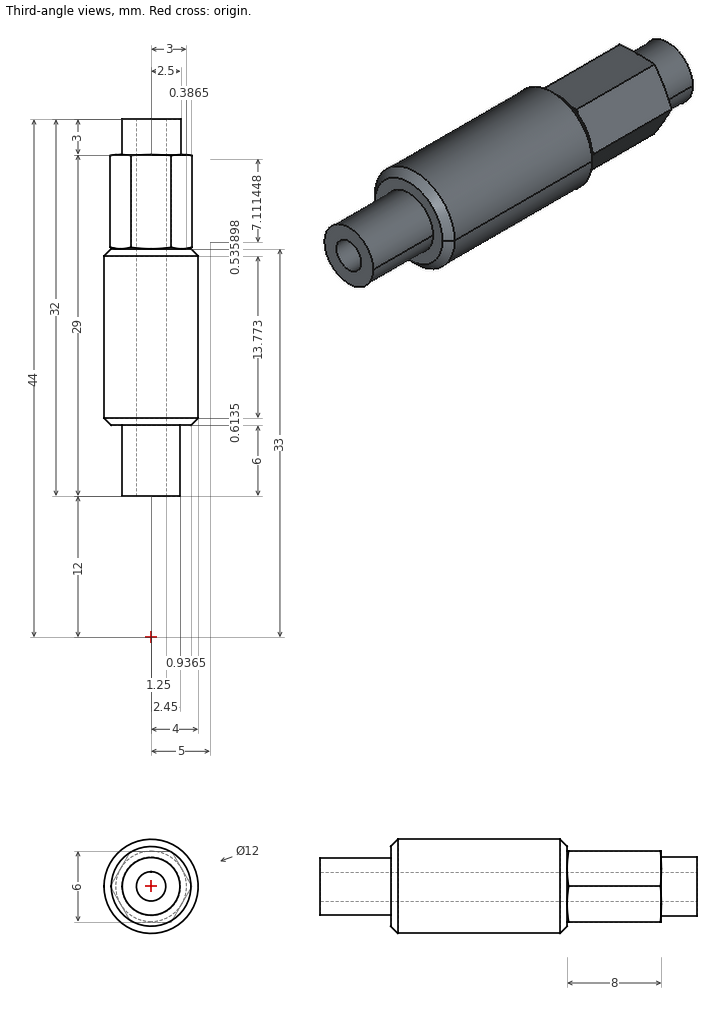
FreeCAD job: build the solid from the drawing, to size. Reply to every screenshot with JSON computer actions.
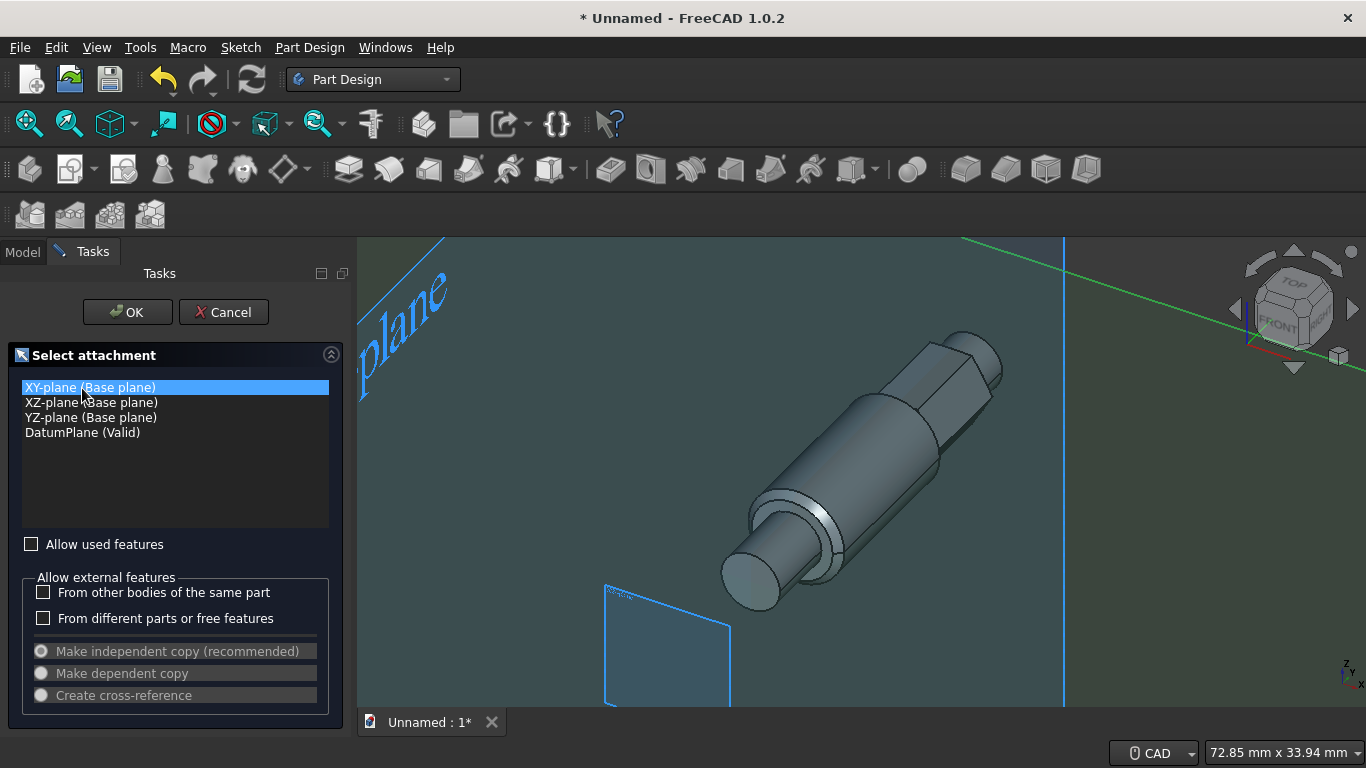
{"action": "left_click", "coordinate": [128, 312]}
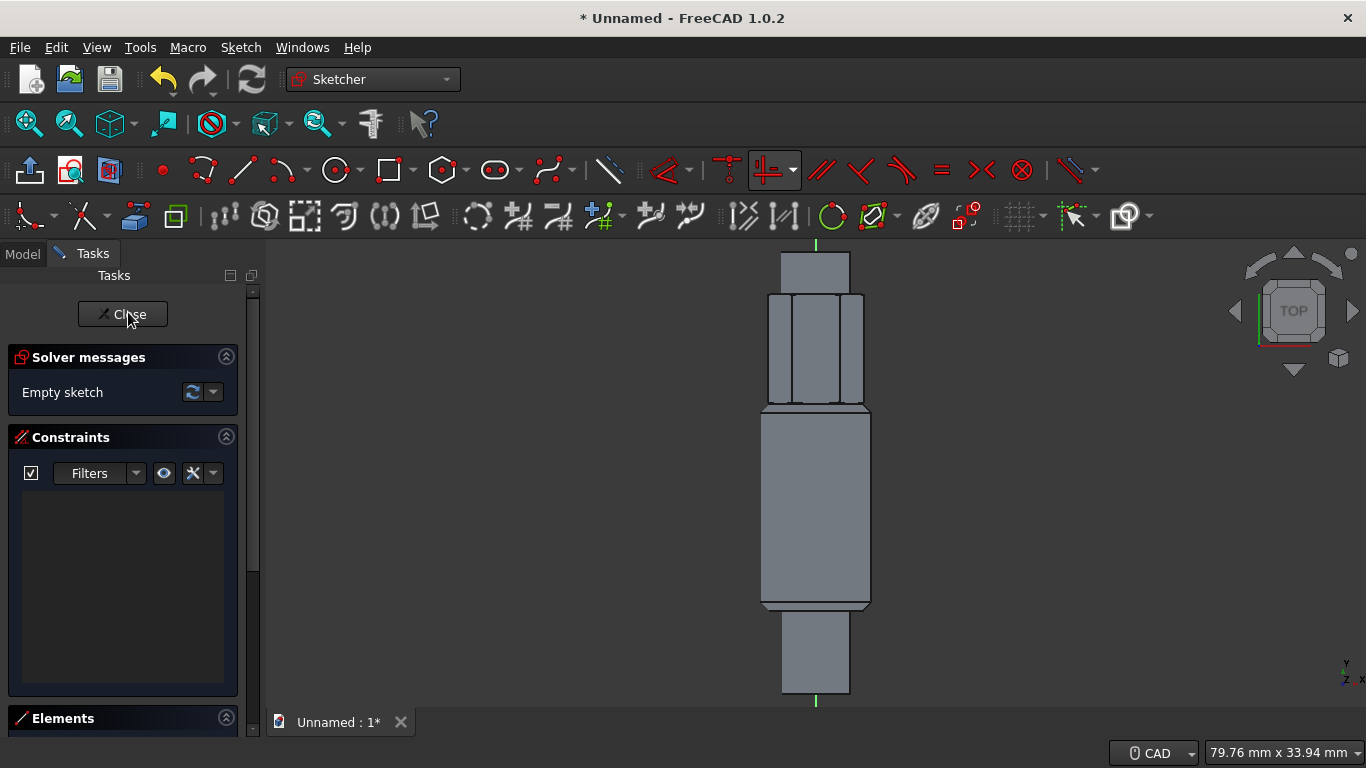
{"action": "left_click", "coordinate": [110, 170]}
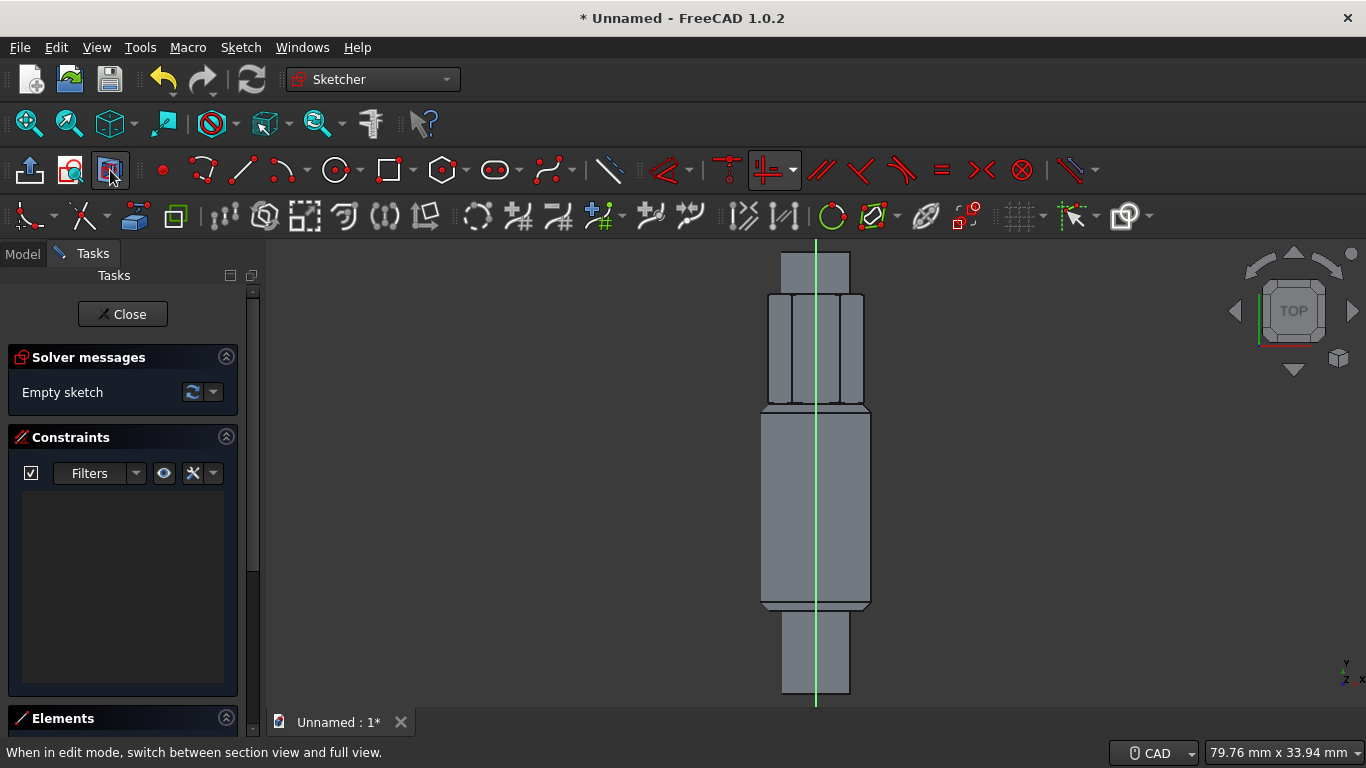
{"action": "scroll", "coordinate": [685, 405], "scroll_direction": "down", "scroll_amount": 4}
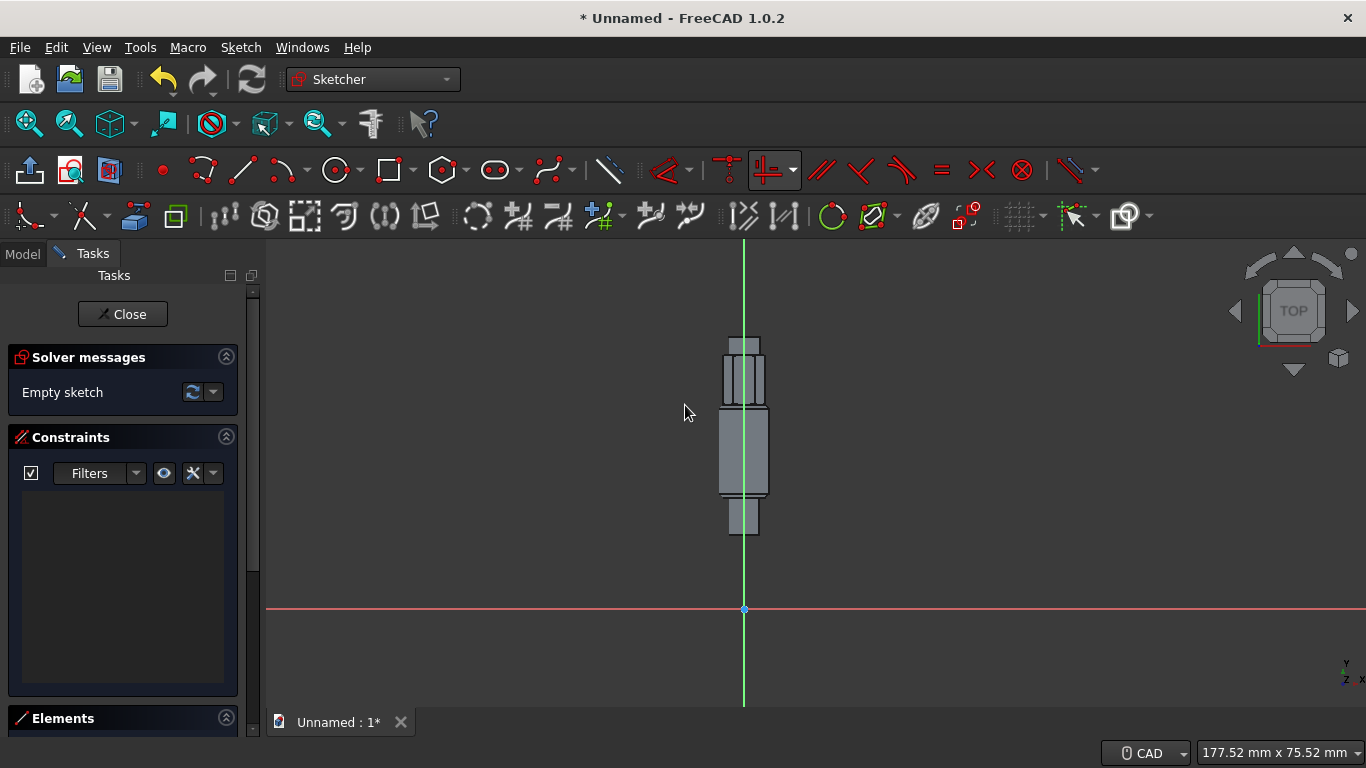
{"action": "left_click", "coordinate": [390, 170]}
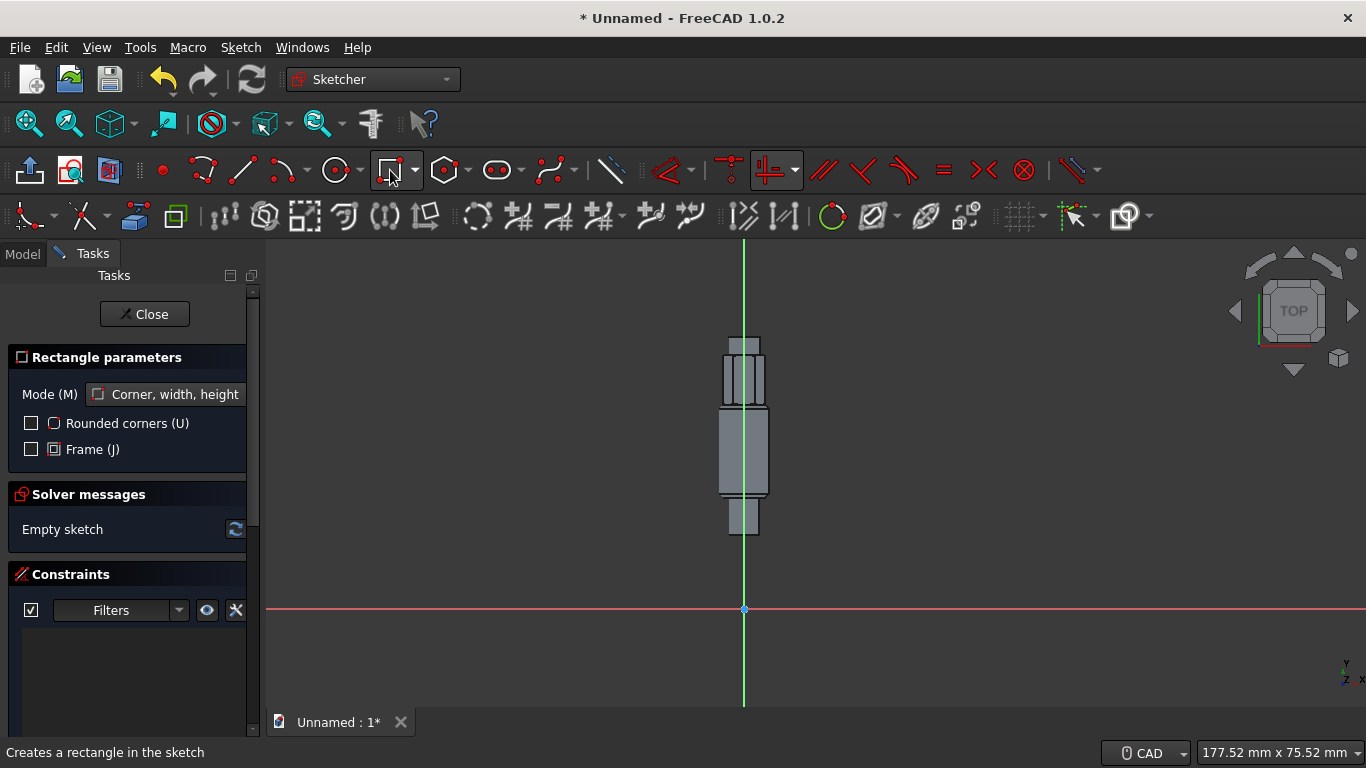
{"action": "scroll", "coordinate": [744, 337], "scroll_direction": "up", "scroll_amount": 4}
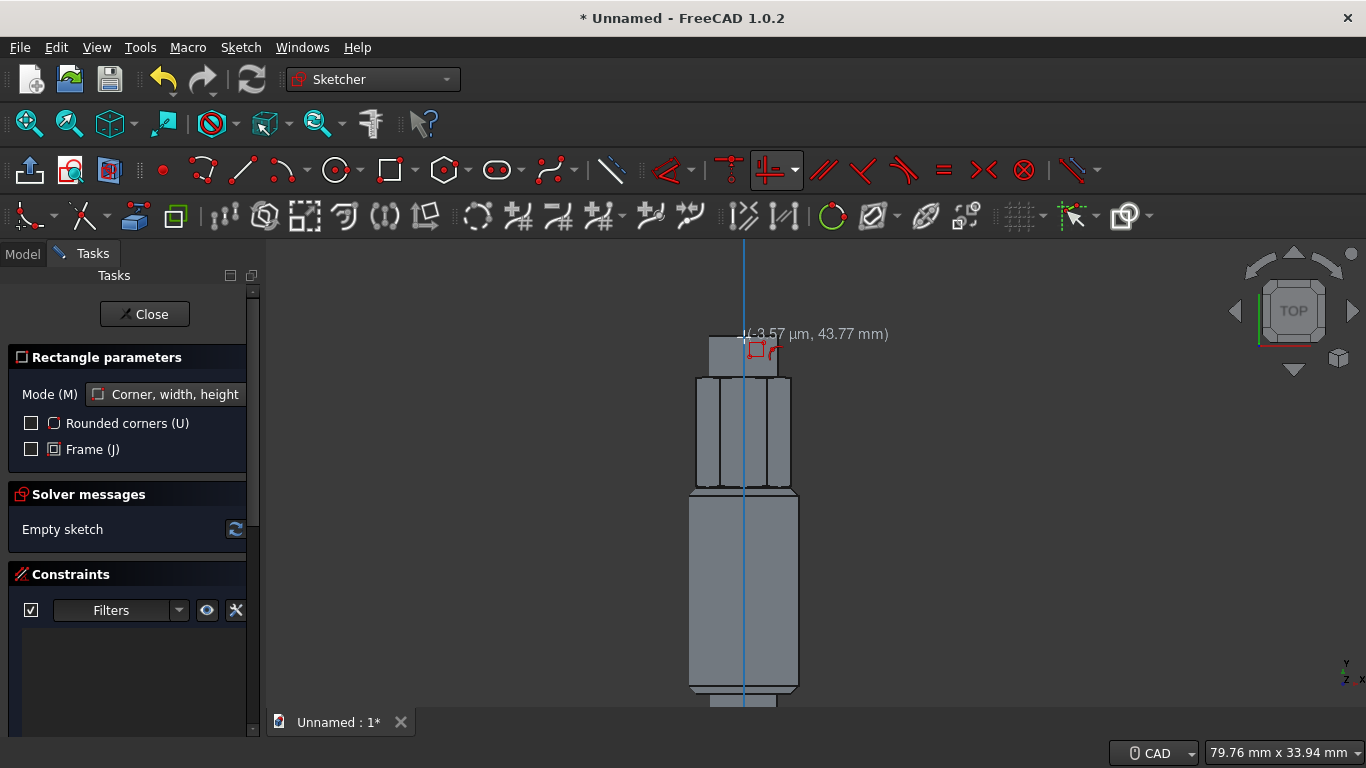
{"action": "left_click", "coordinate": [744, 336]}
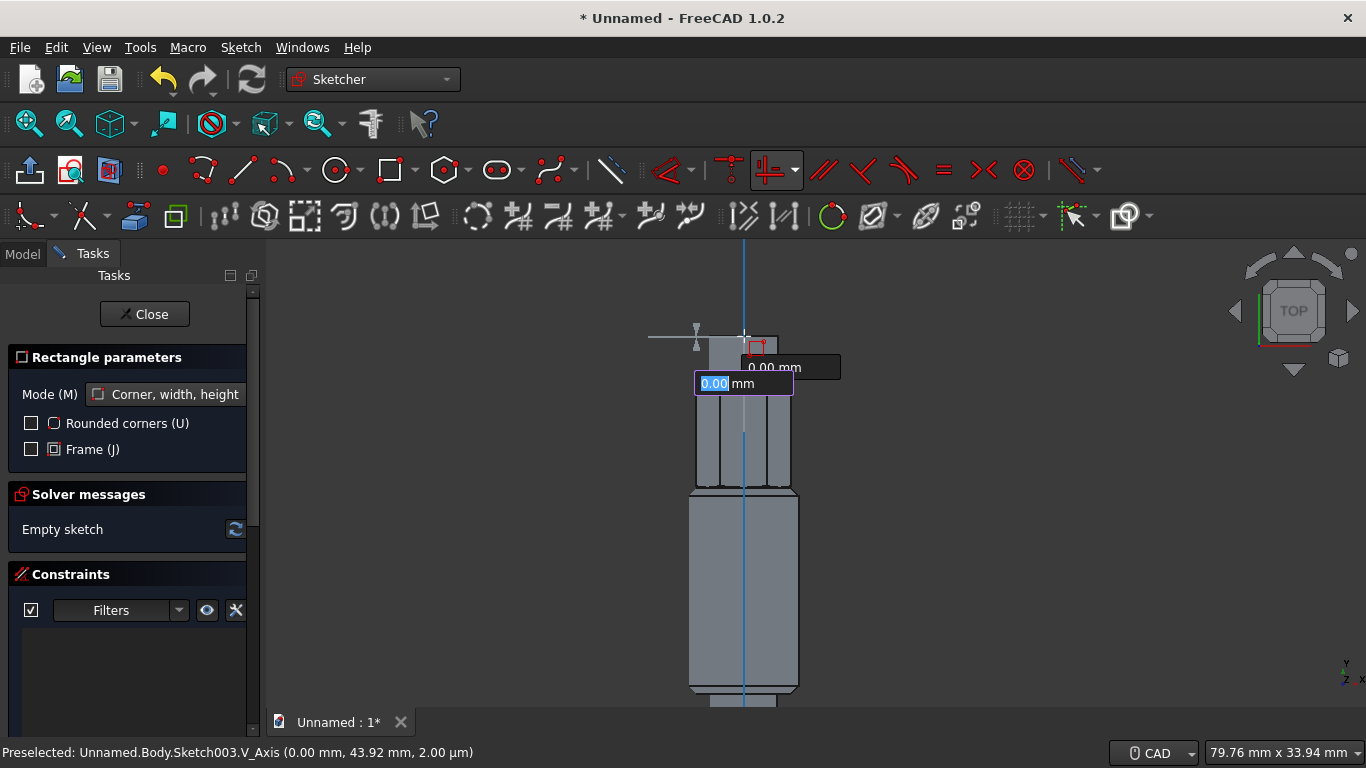
{"action": "scroll", "coordinate": [744, 337], "scroll_direction": "down", "scroll_amount": 4}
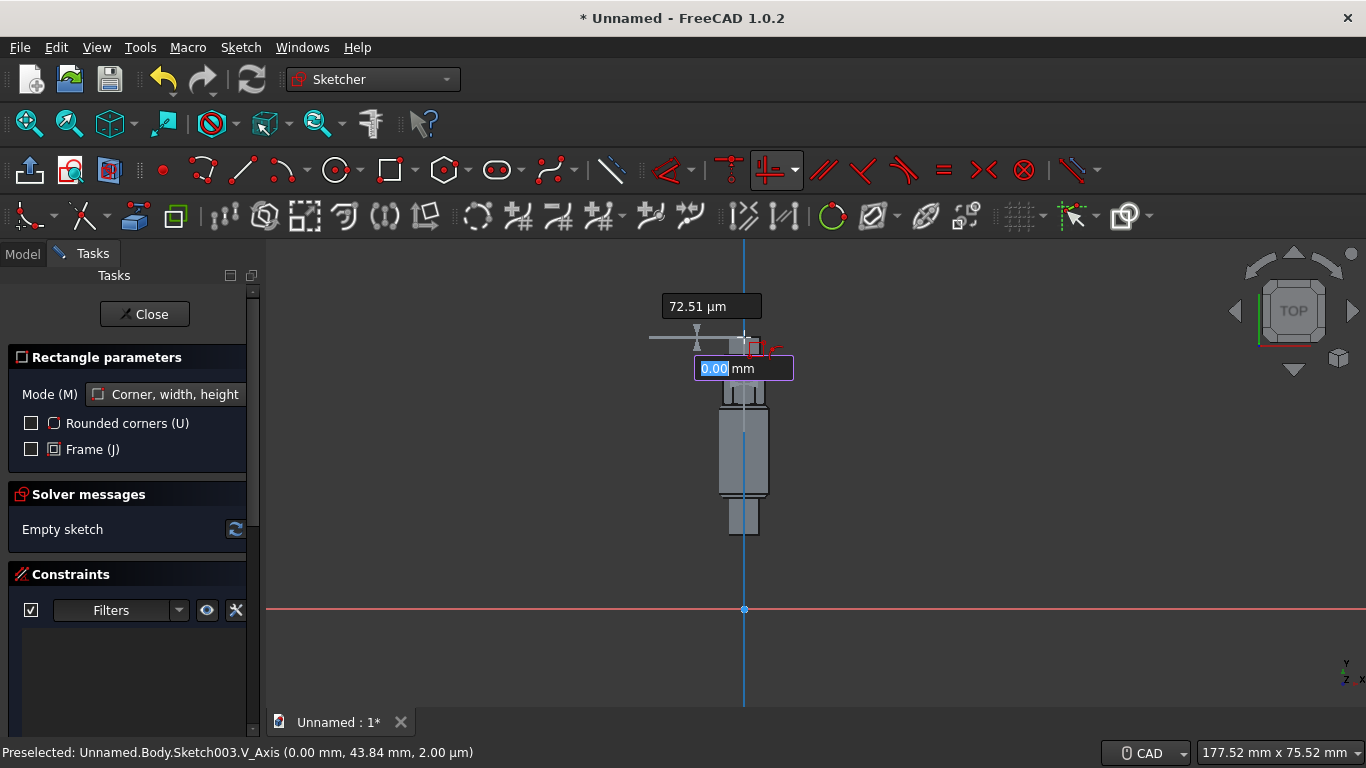
{"action": "scroll", "coordinate": [752, 535], "scroll_direction": "up", "scroll_amount": 4}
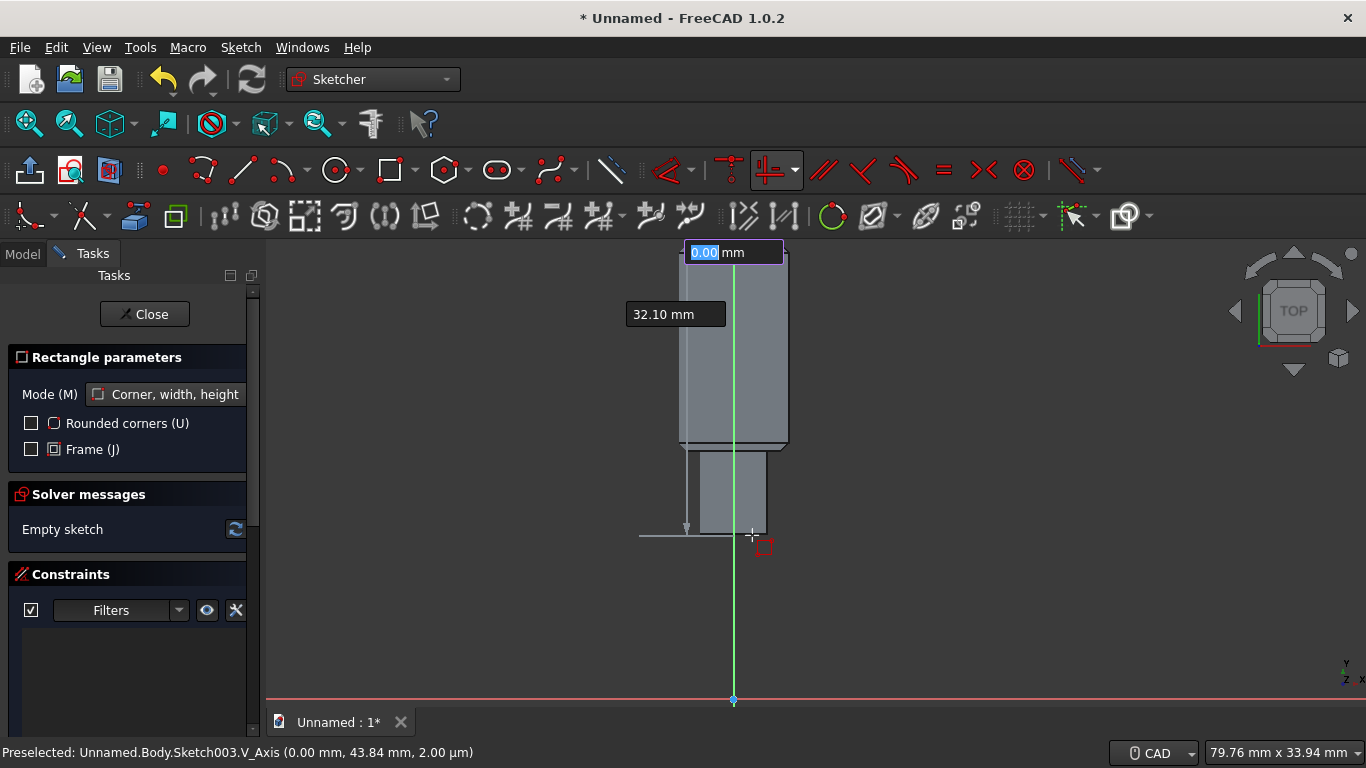
{"action": "left_click", "coordinate": [751, 534]}
{"action": "key", "text": "Escape"}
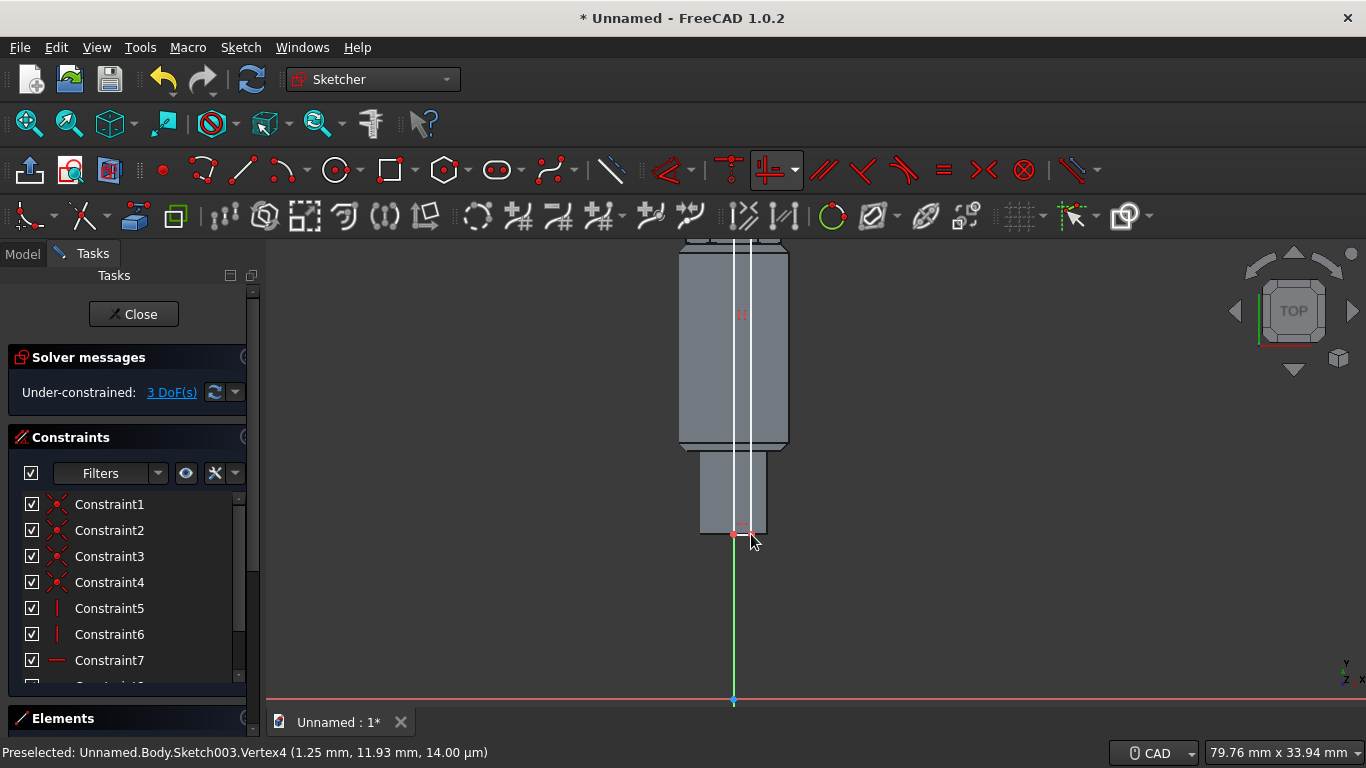
{"action": "left_click", "coordinate": [666, 170]}